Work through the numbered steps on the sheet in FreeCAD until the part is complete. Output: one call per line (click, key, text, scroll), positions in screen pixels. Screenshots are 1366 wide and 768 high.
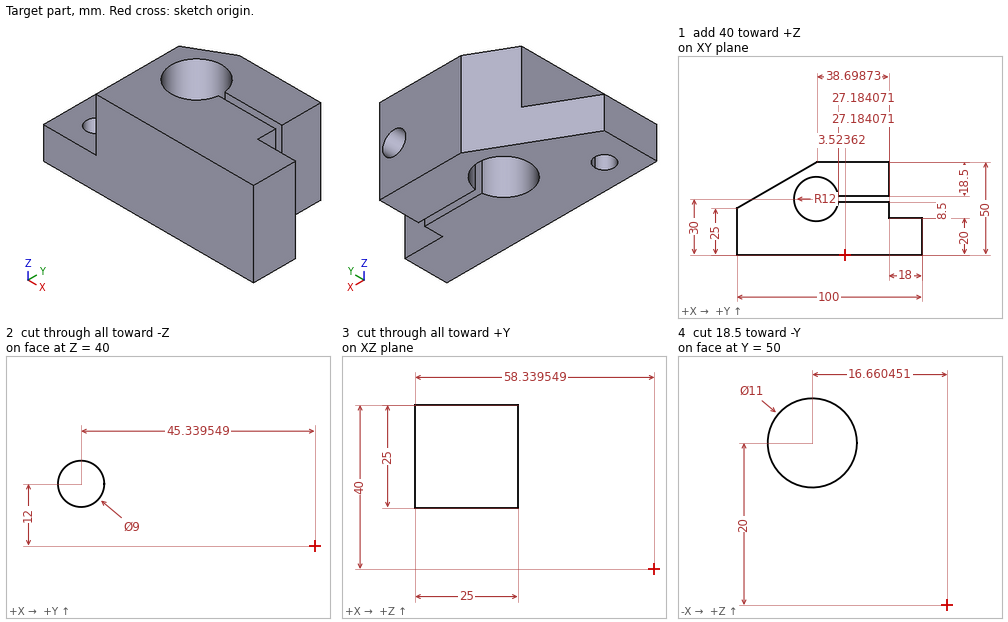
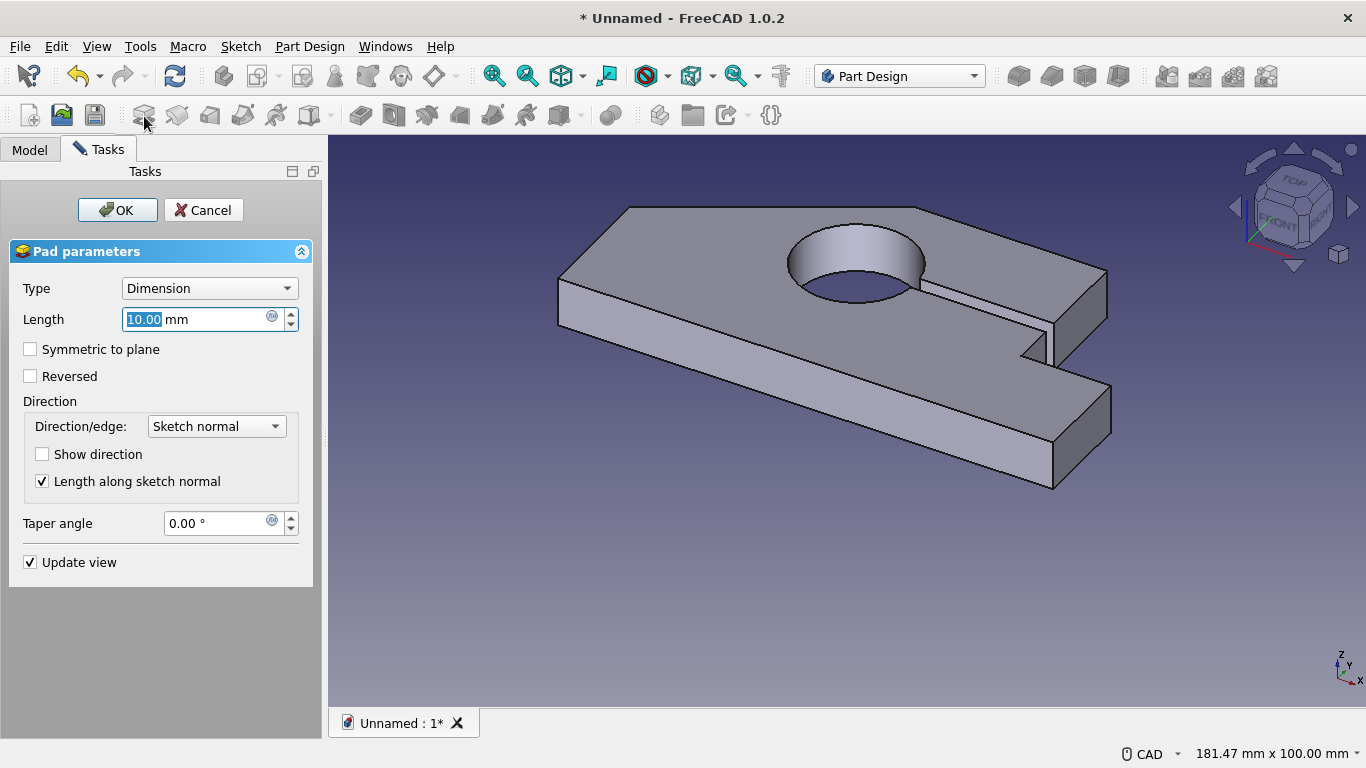
text(40)
key(Tab)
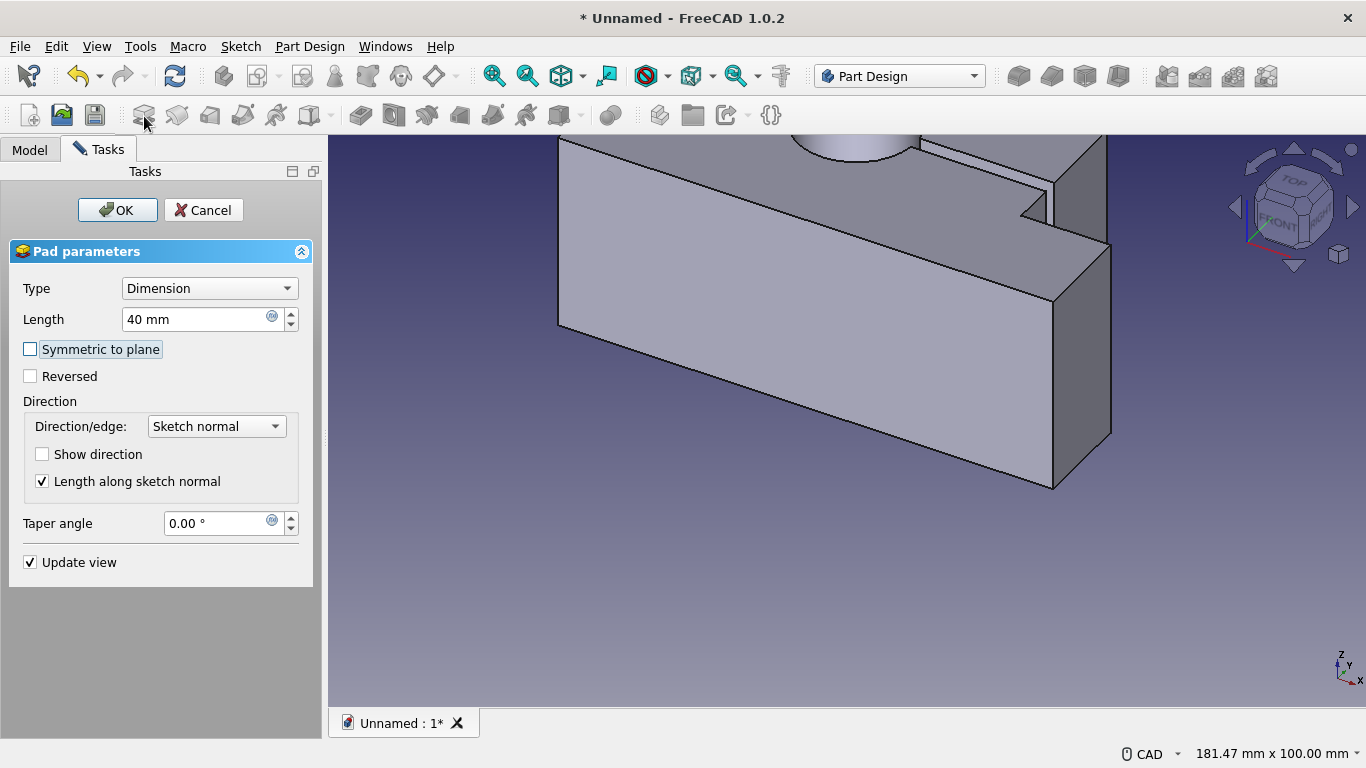
click(118, 210)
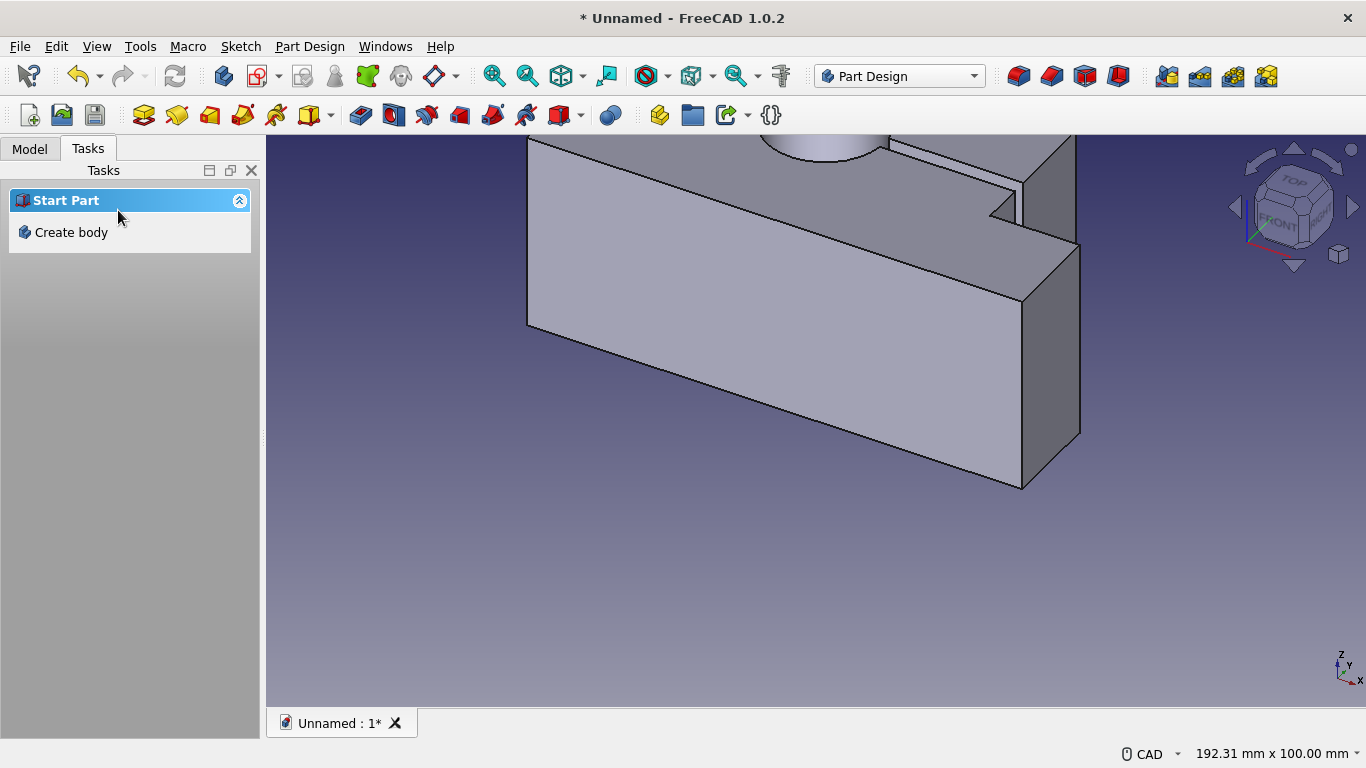
click(495, 76)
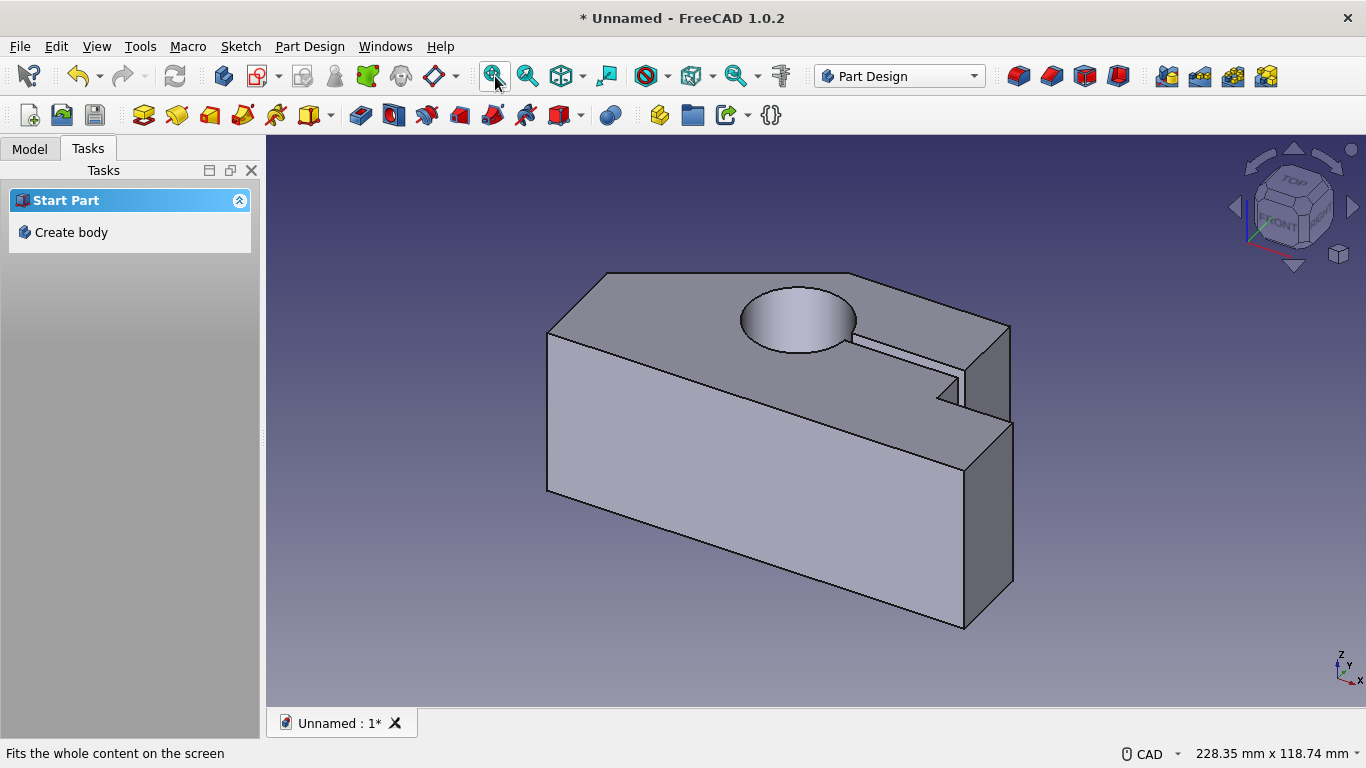
click(680, 319)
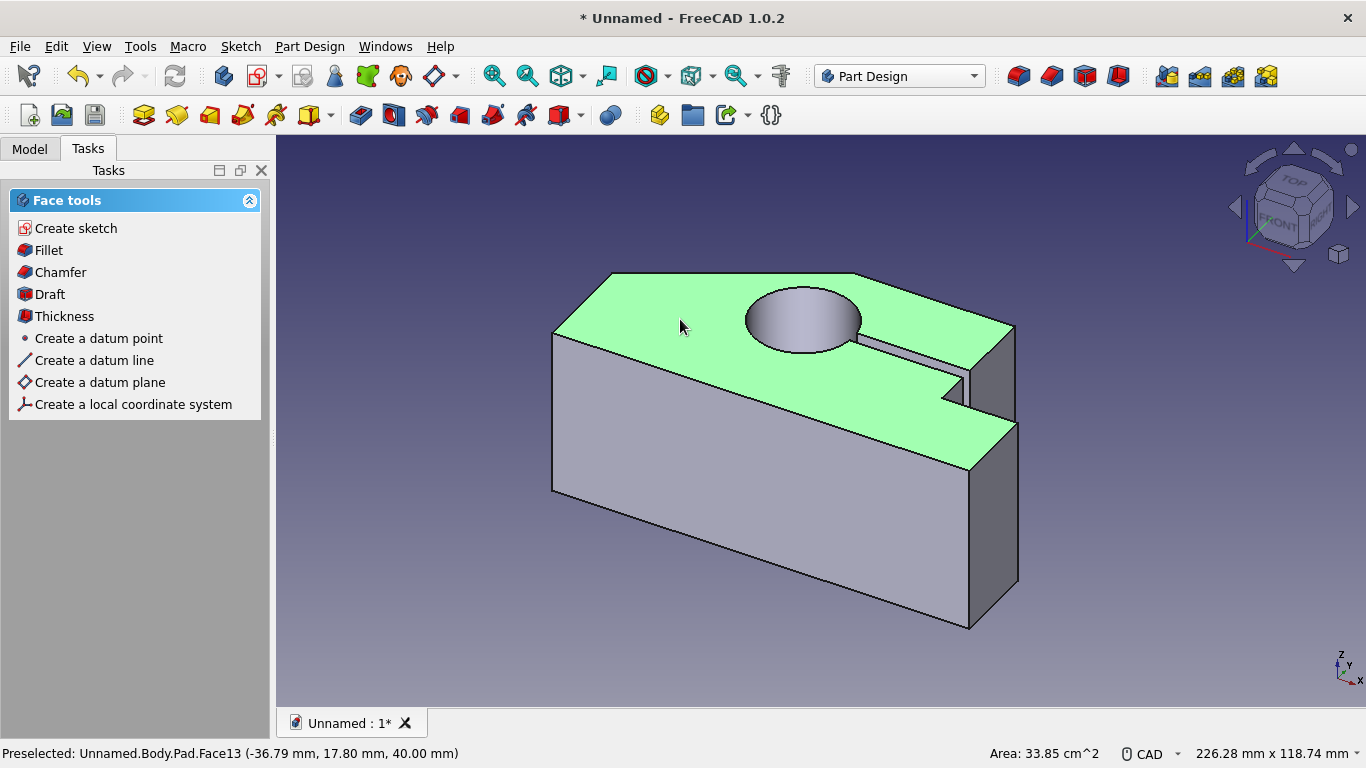
click(256, 76)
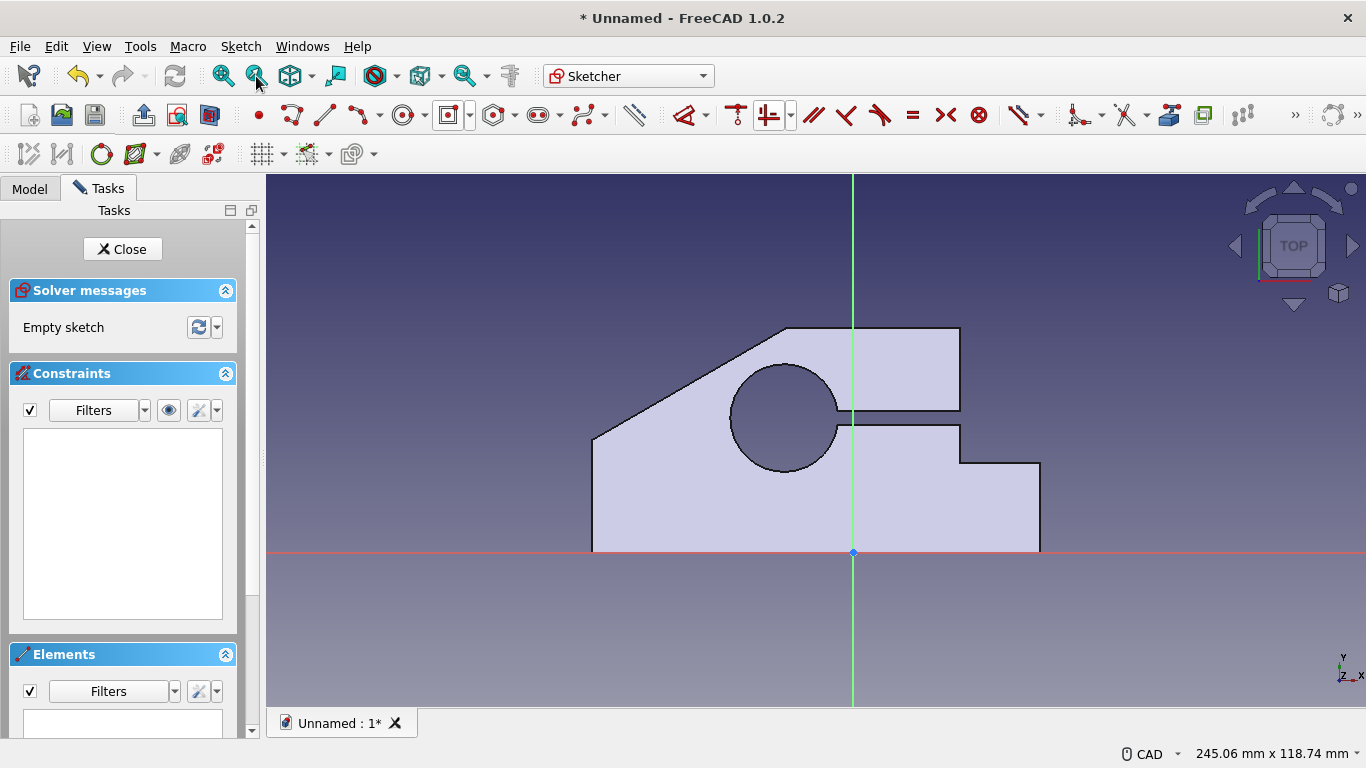
scroll(638, 506, up, 11)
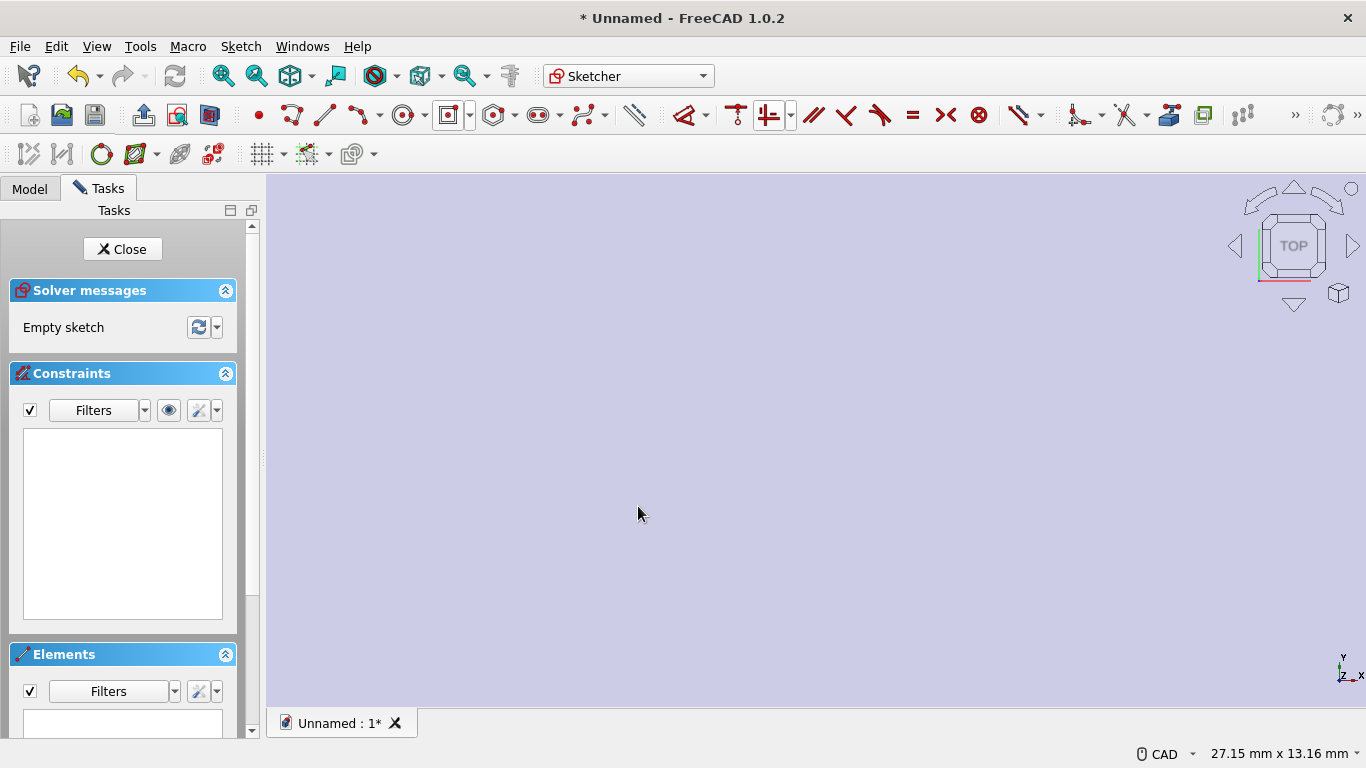
click(402, 116)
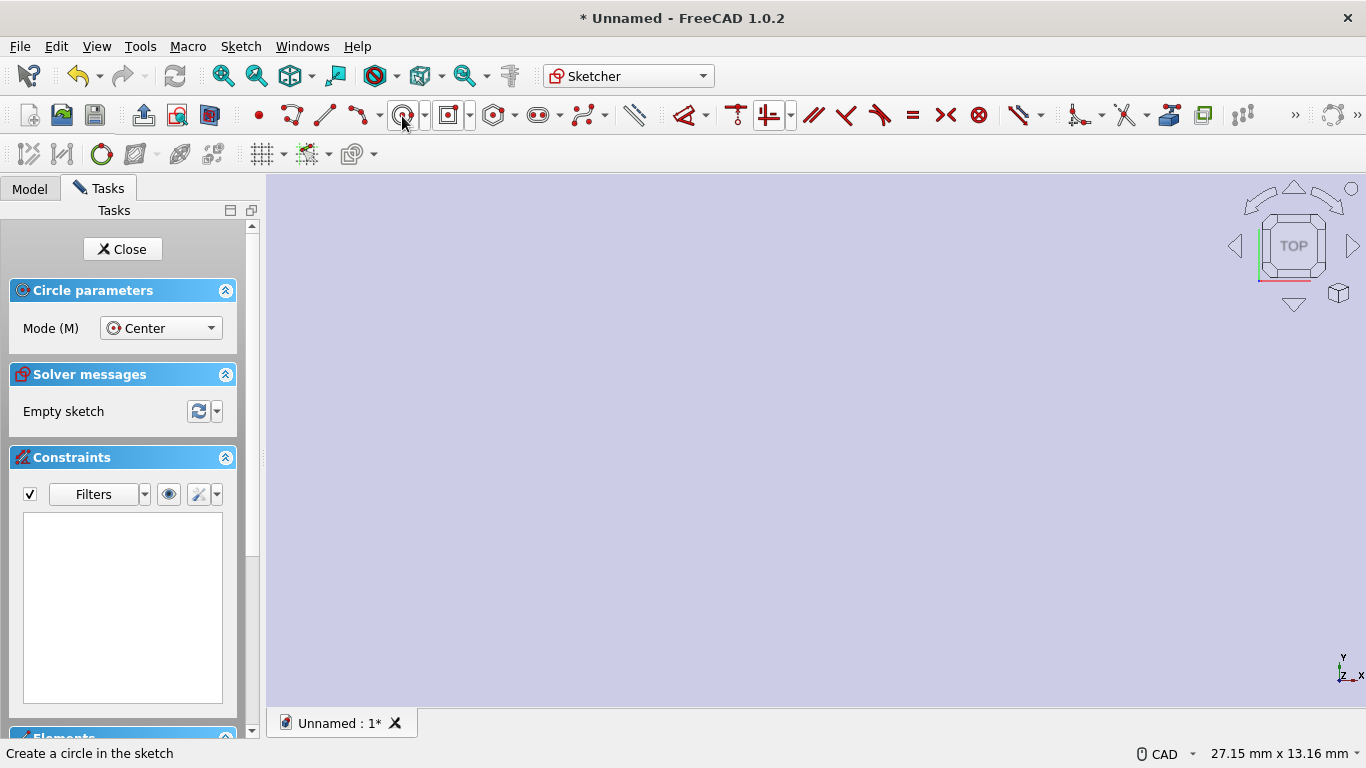
click(743, 436)
move(872, 308)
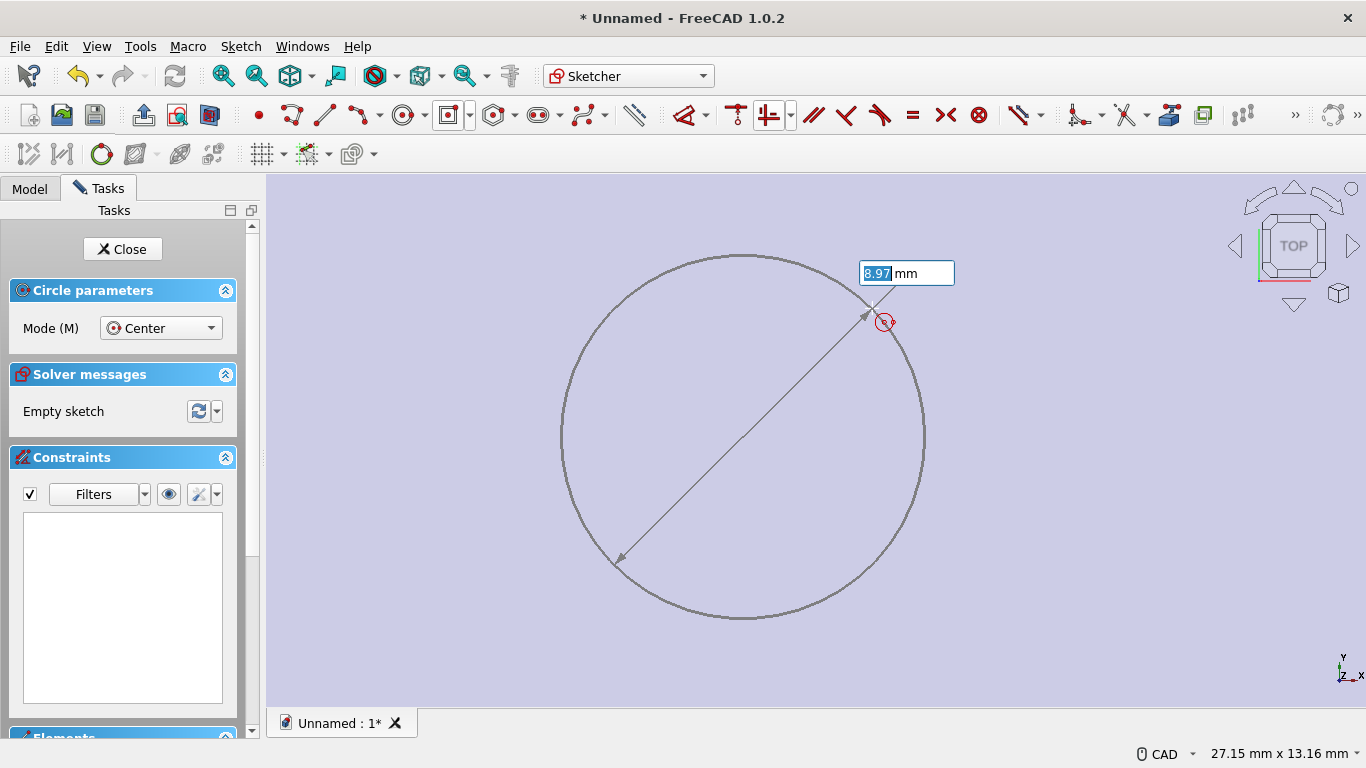
text(9)
key(Return)
key(Escape)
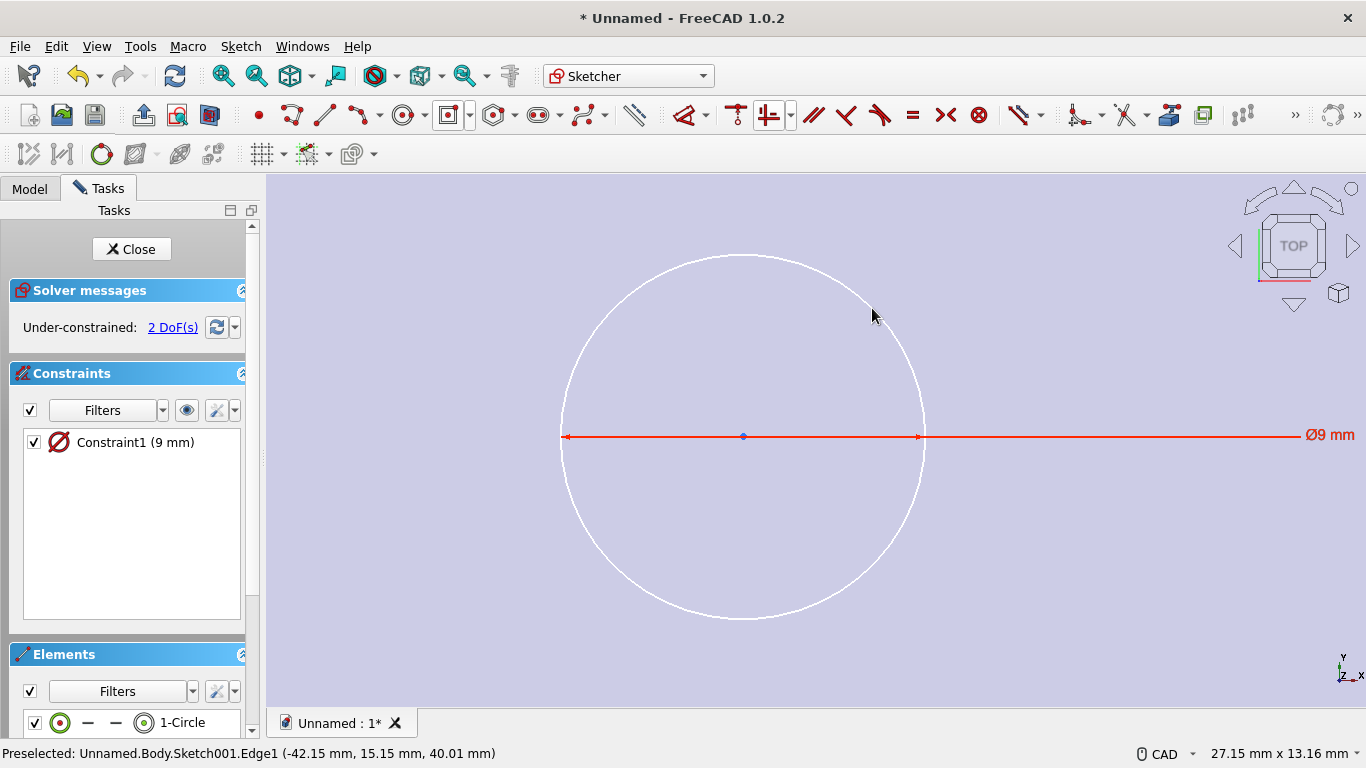
key(d)